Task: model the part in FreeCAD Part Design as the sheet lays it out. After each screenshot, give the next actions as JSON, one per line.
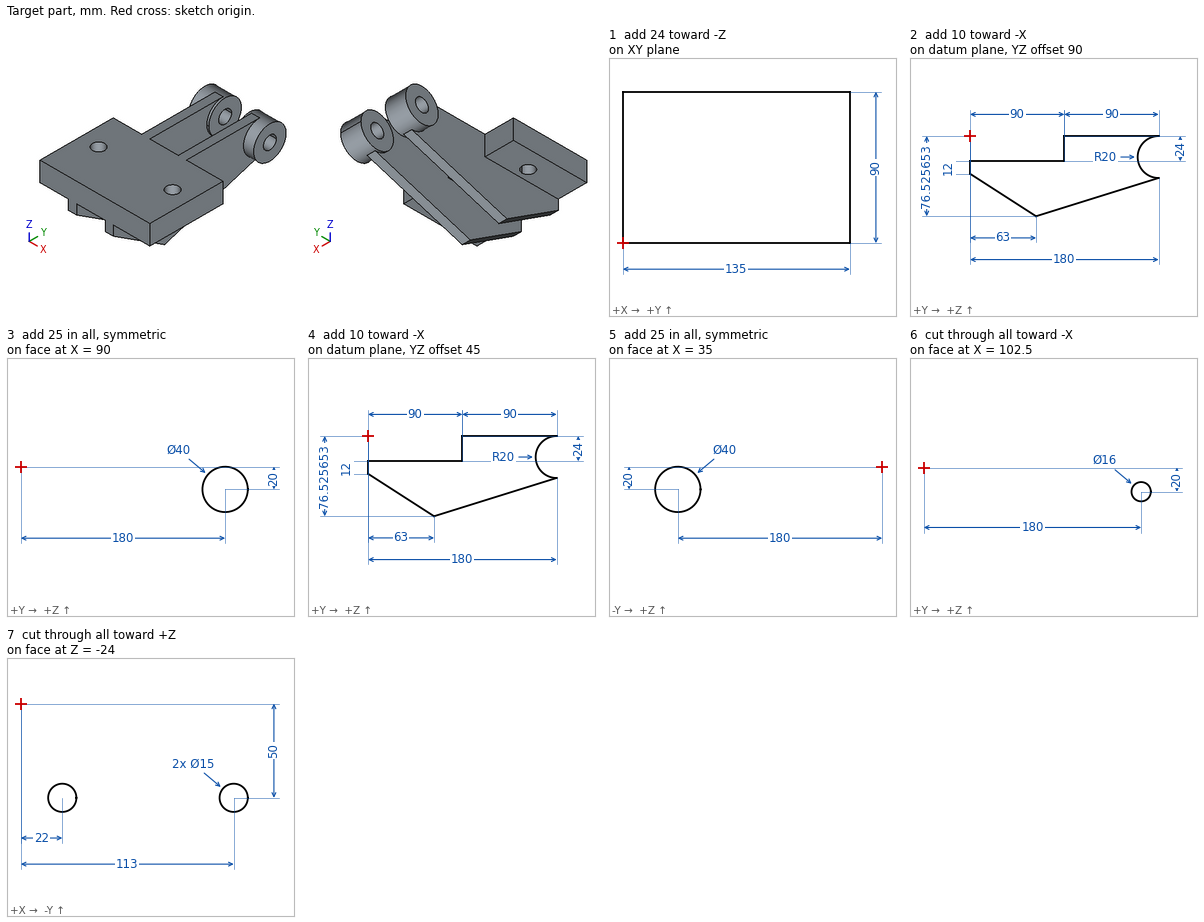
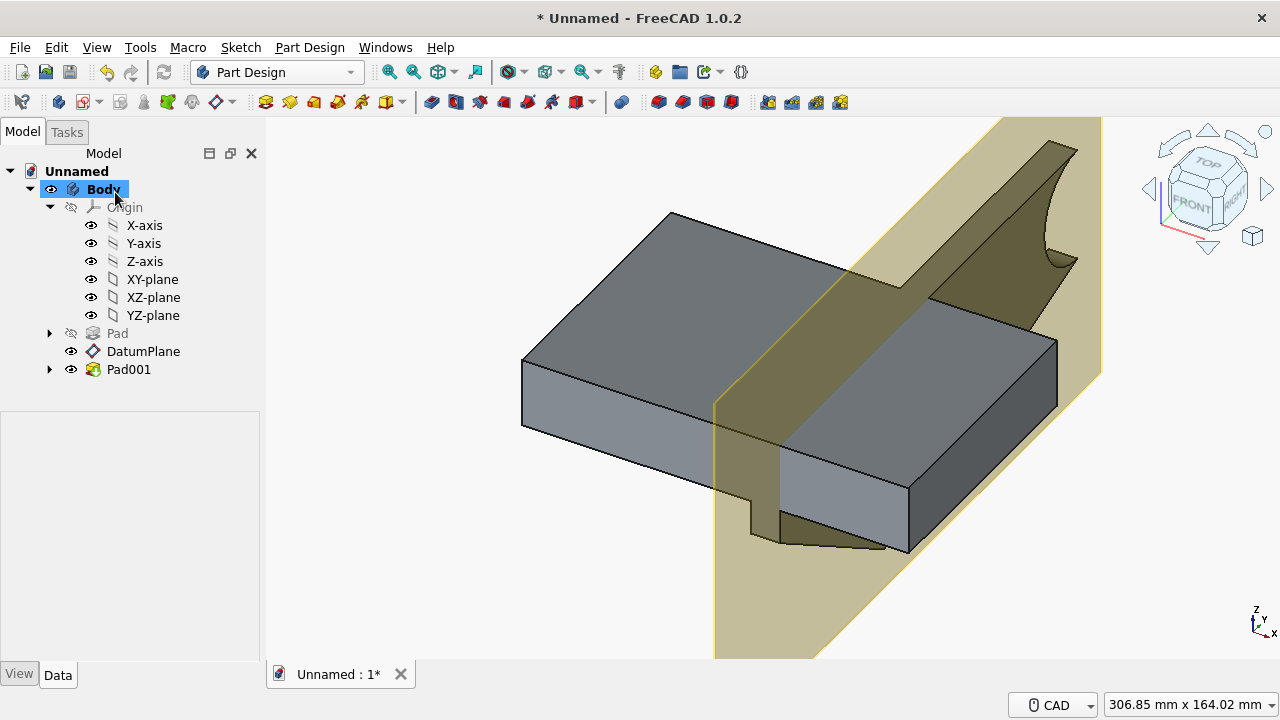
{"action": "left_click", "coordinate": [116, 351]}
{"action": "key", "text": "space"}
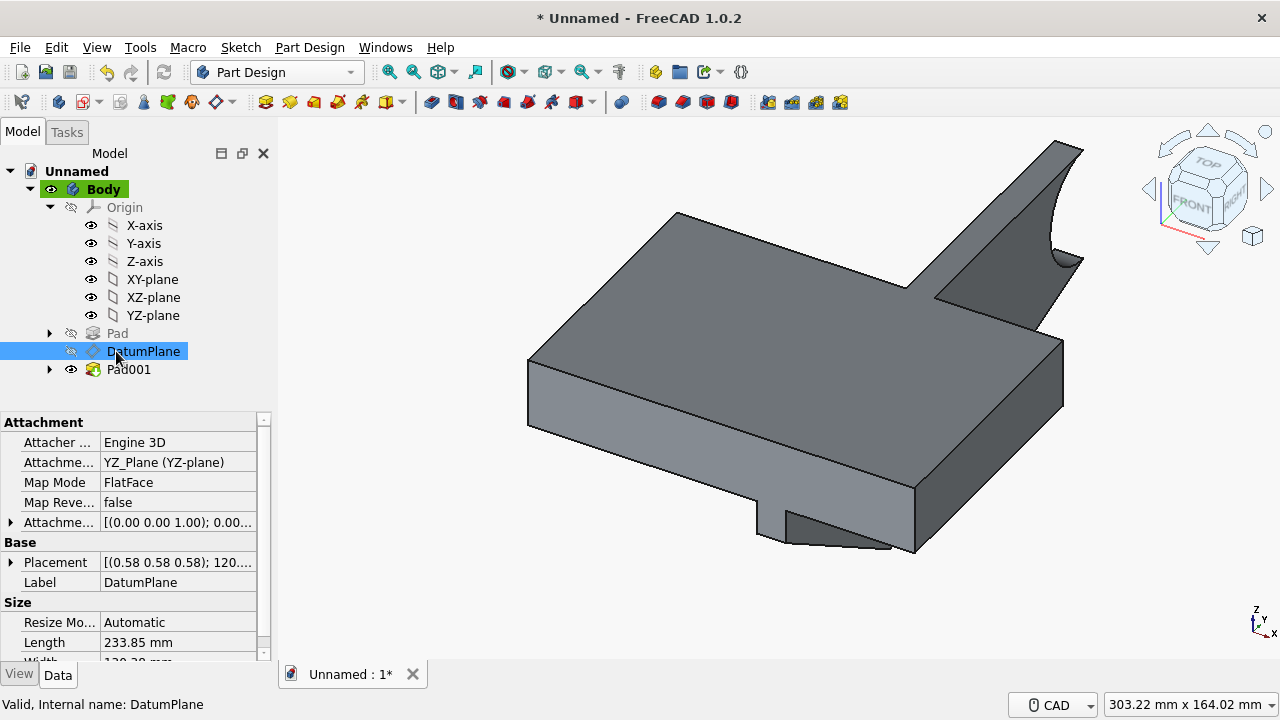
{"action": "left_click", "coordinate": [390, 72]}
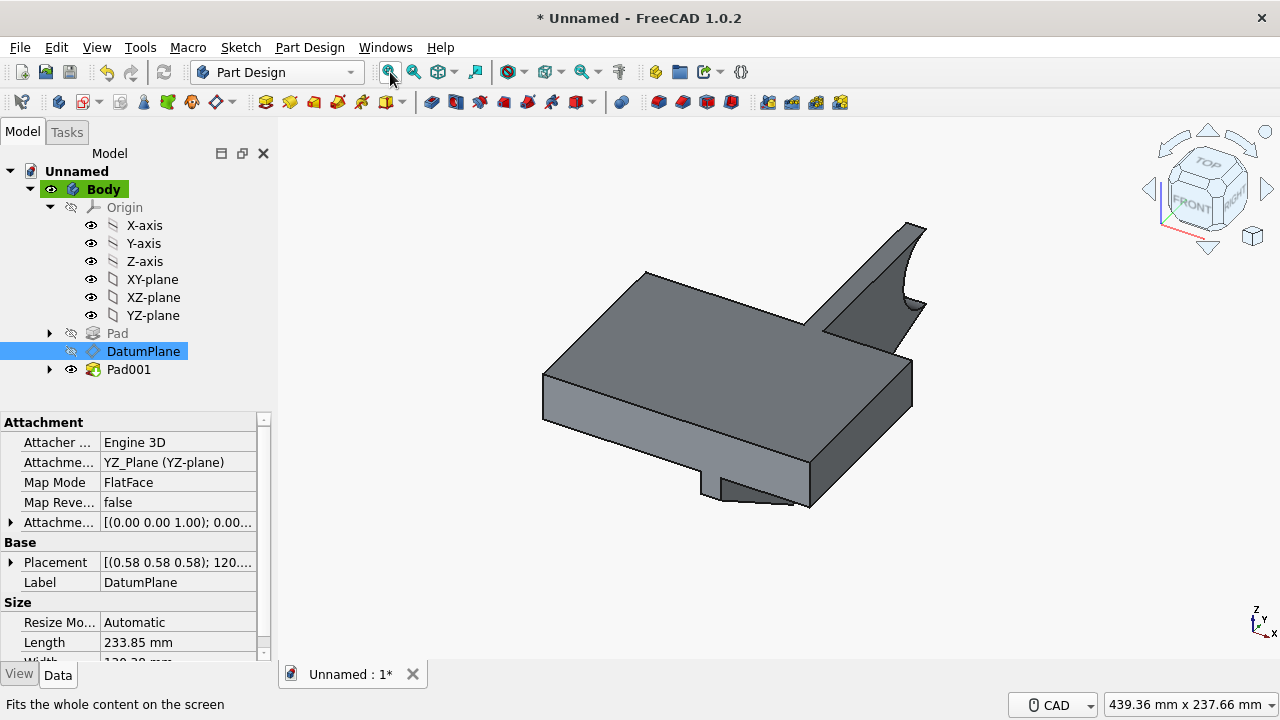
{"action": "left_click", "coordinate": [882, 323]}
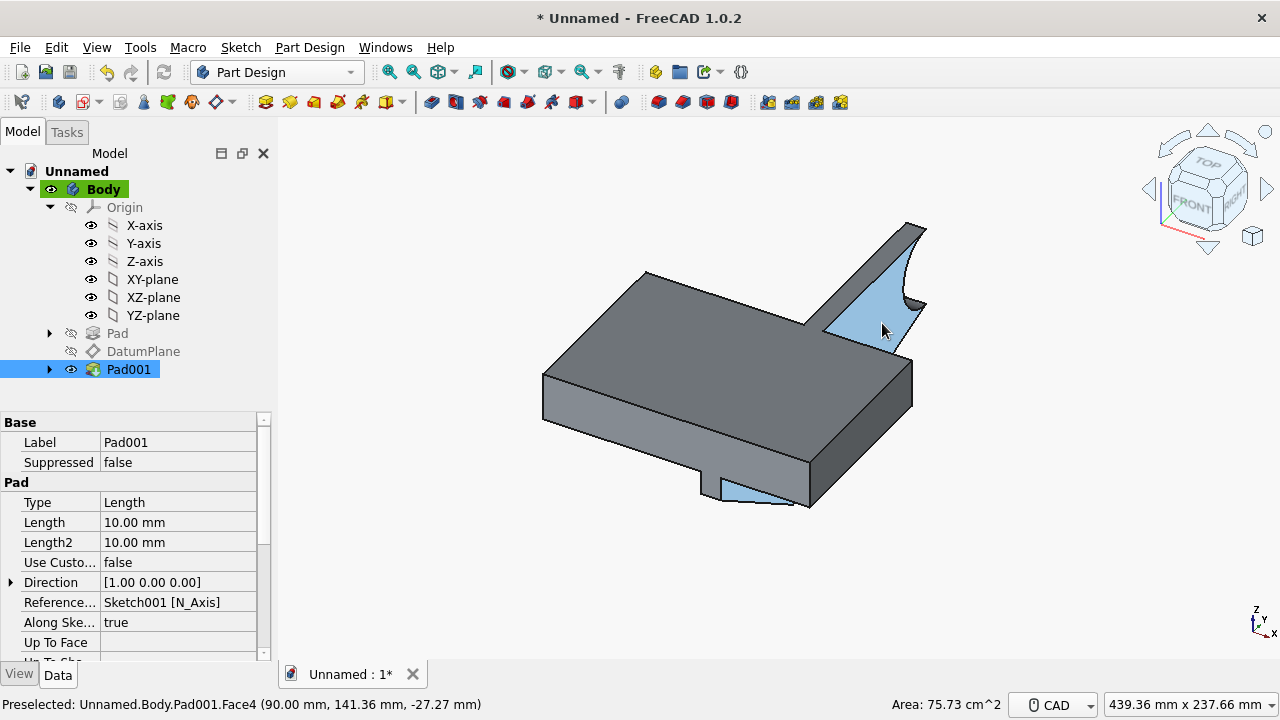
{"action": "left_click", "coordinate": [84, 102]}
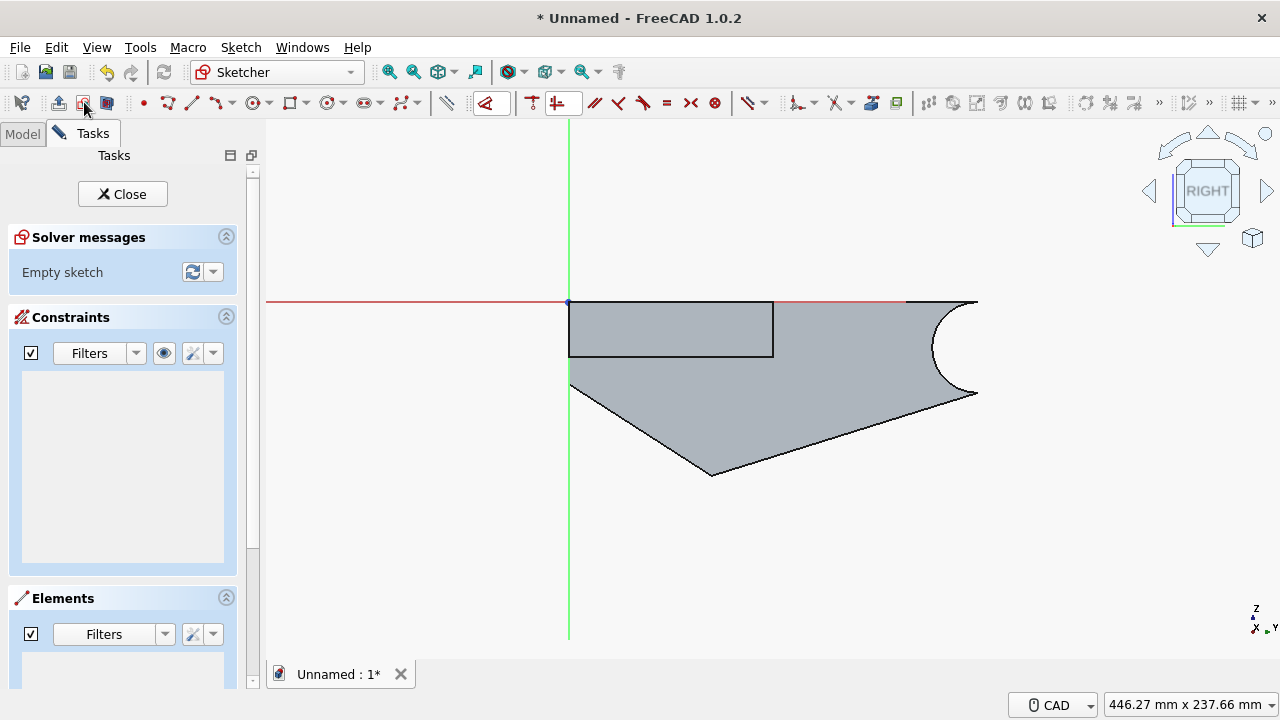
{"action": "left_click", "coordinate": [108, 104]}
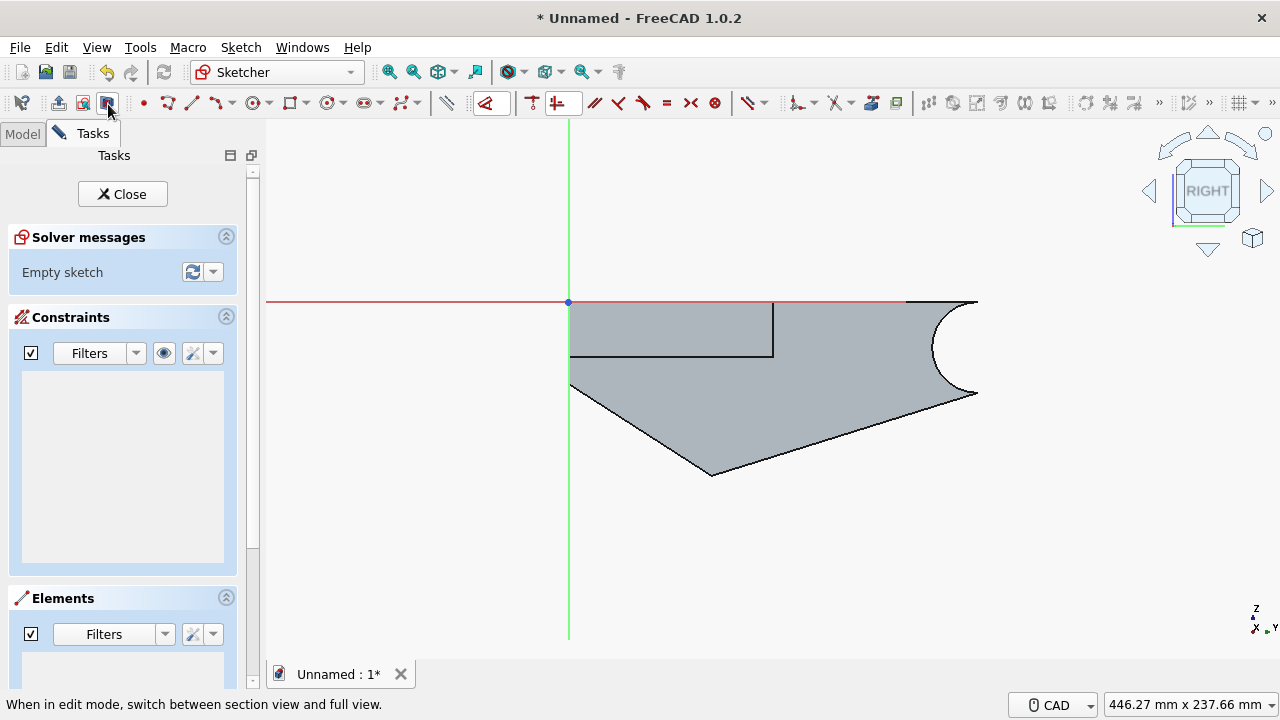
{"action": "scroll", "coordinate": [1067, 334], "scroll_direction": "up", "scroll_amount": 7}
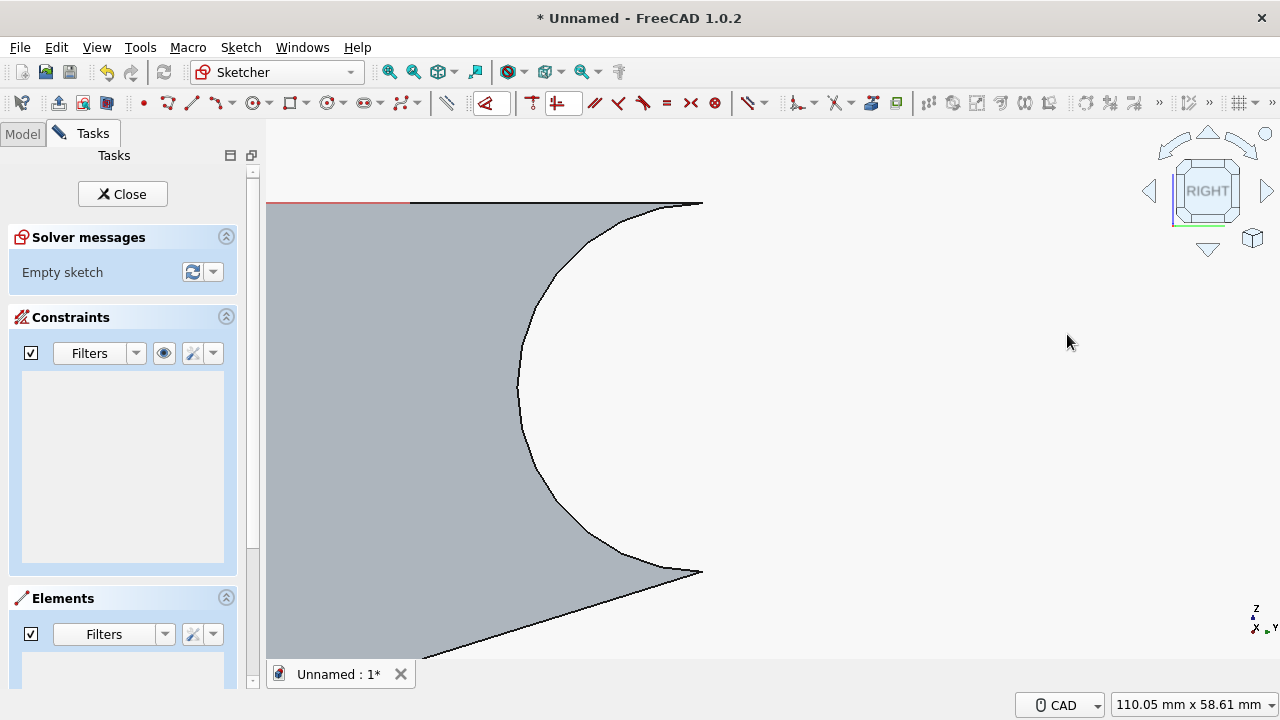
{"action": "left_click", "coordinate": [254, 104]}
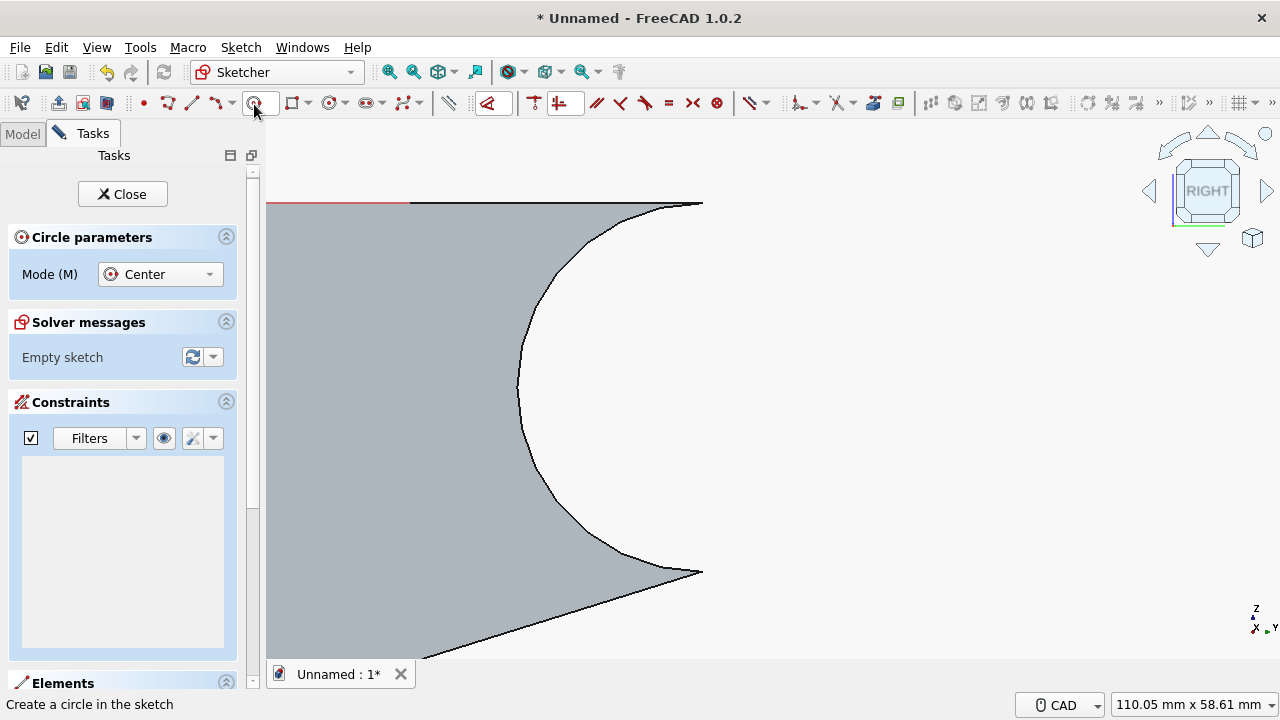
{"action": "left_click", "coordinate": [702, 388]}
{"action": "mouse_move", "coordinate": [832, 257]}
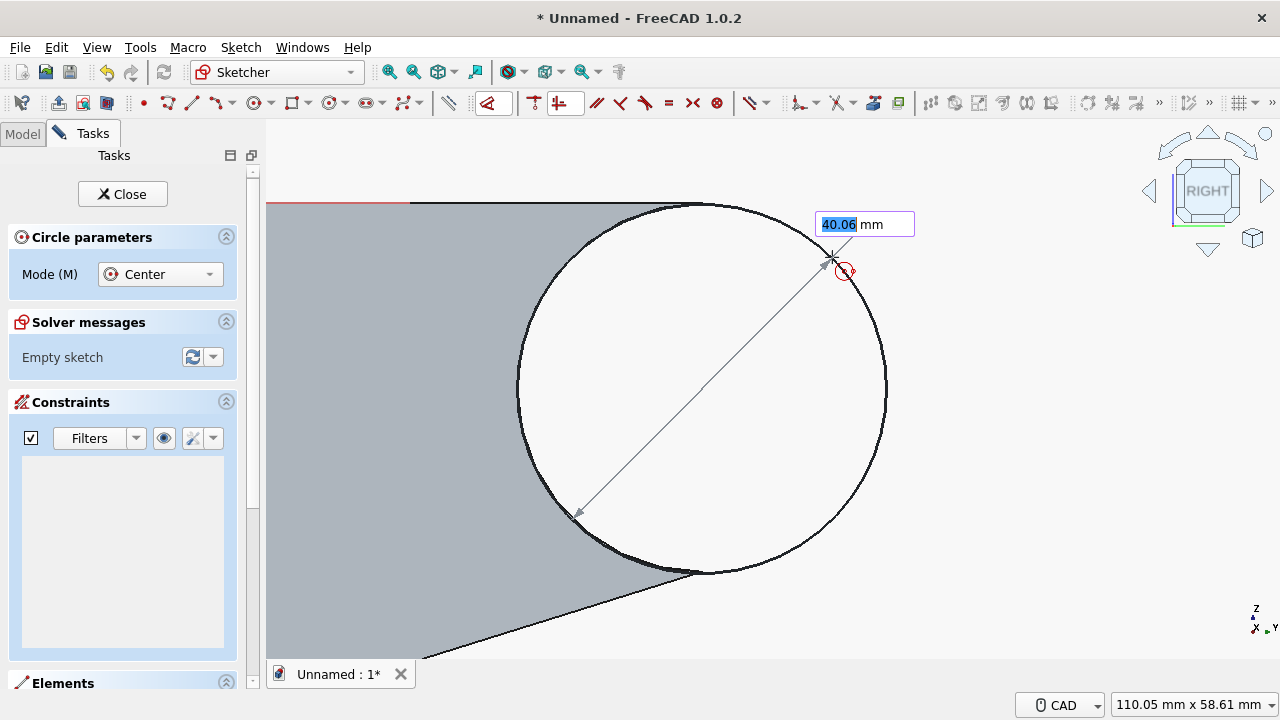
{"action": "type", "text": "40"}
{"action": "key", "text": "Return"}
{"action": "key", "text": "Escape"}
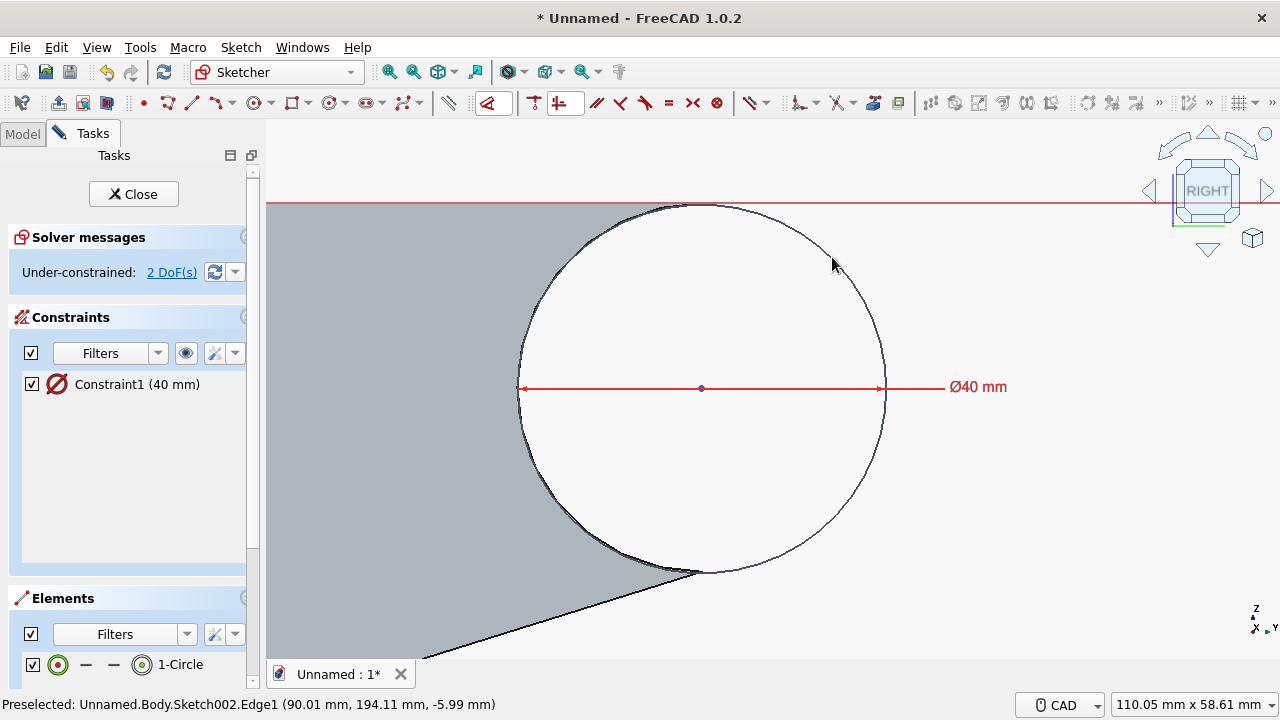
{"action": "left_click", "coordinate": [702, 389]}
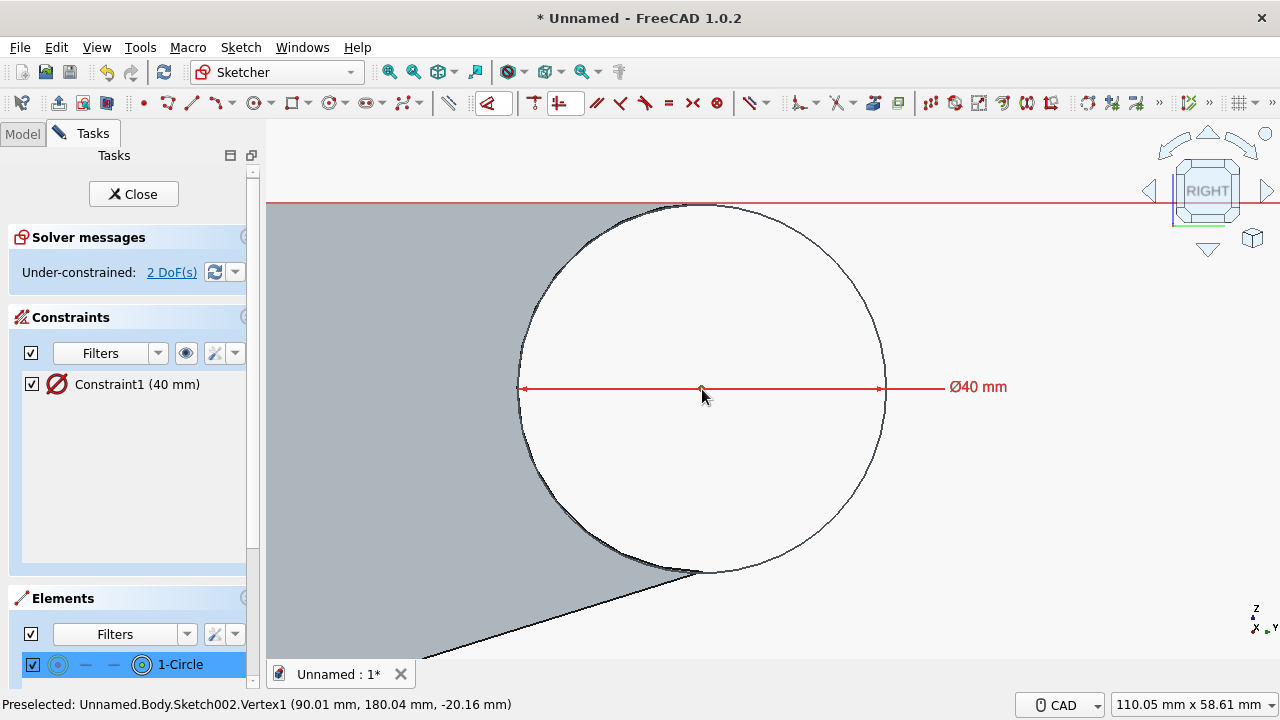
{"action": "left_click", "coordinate": [506, 104]}